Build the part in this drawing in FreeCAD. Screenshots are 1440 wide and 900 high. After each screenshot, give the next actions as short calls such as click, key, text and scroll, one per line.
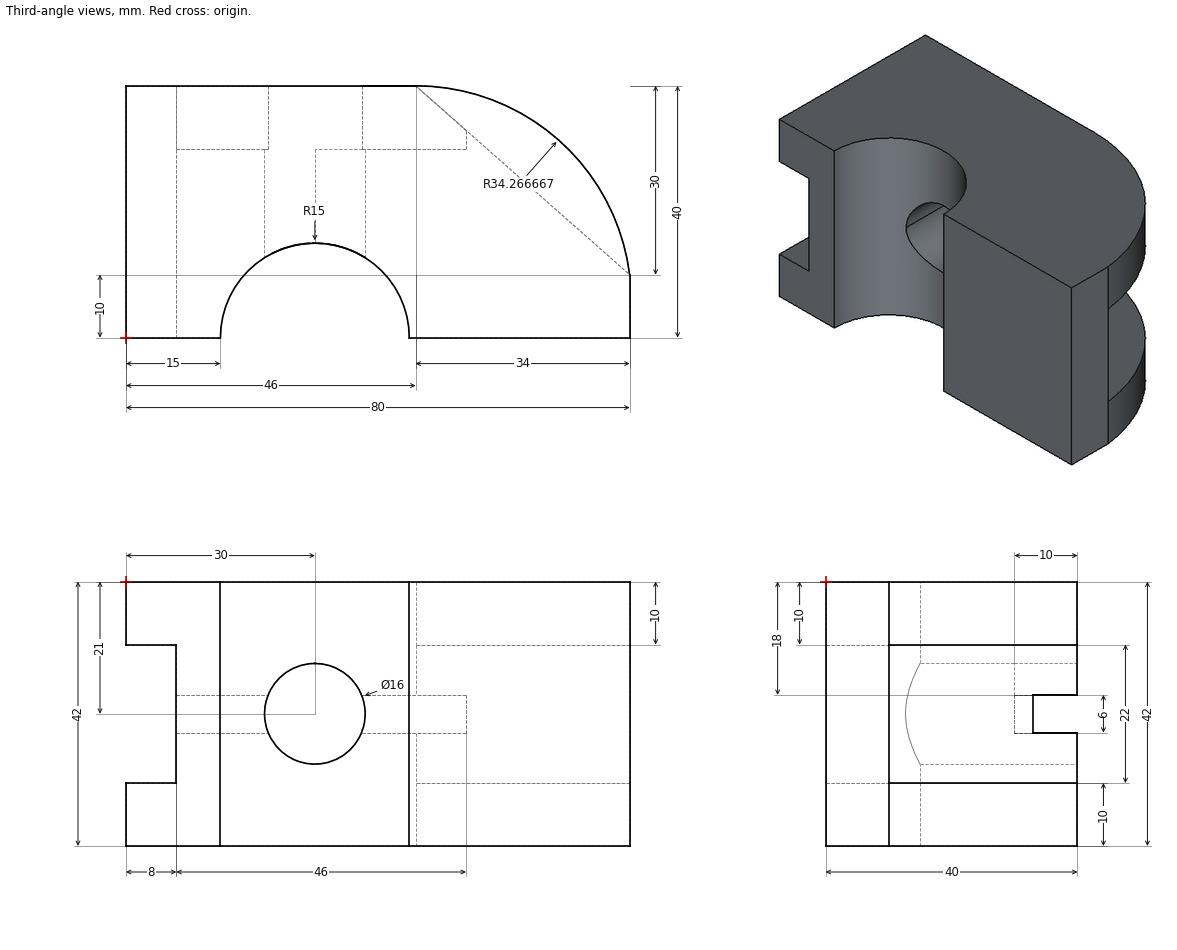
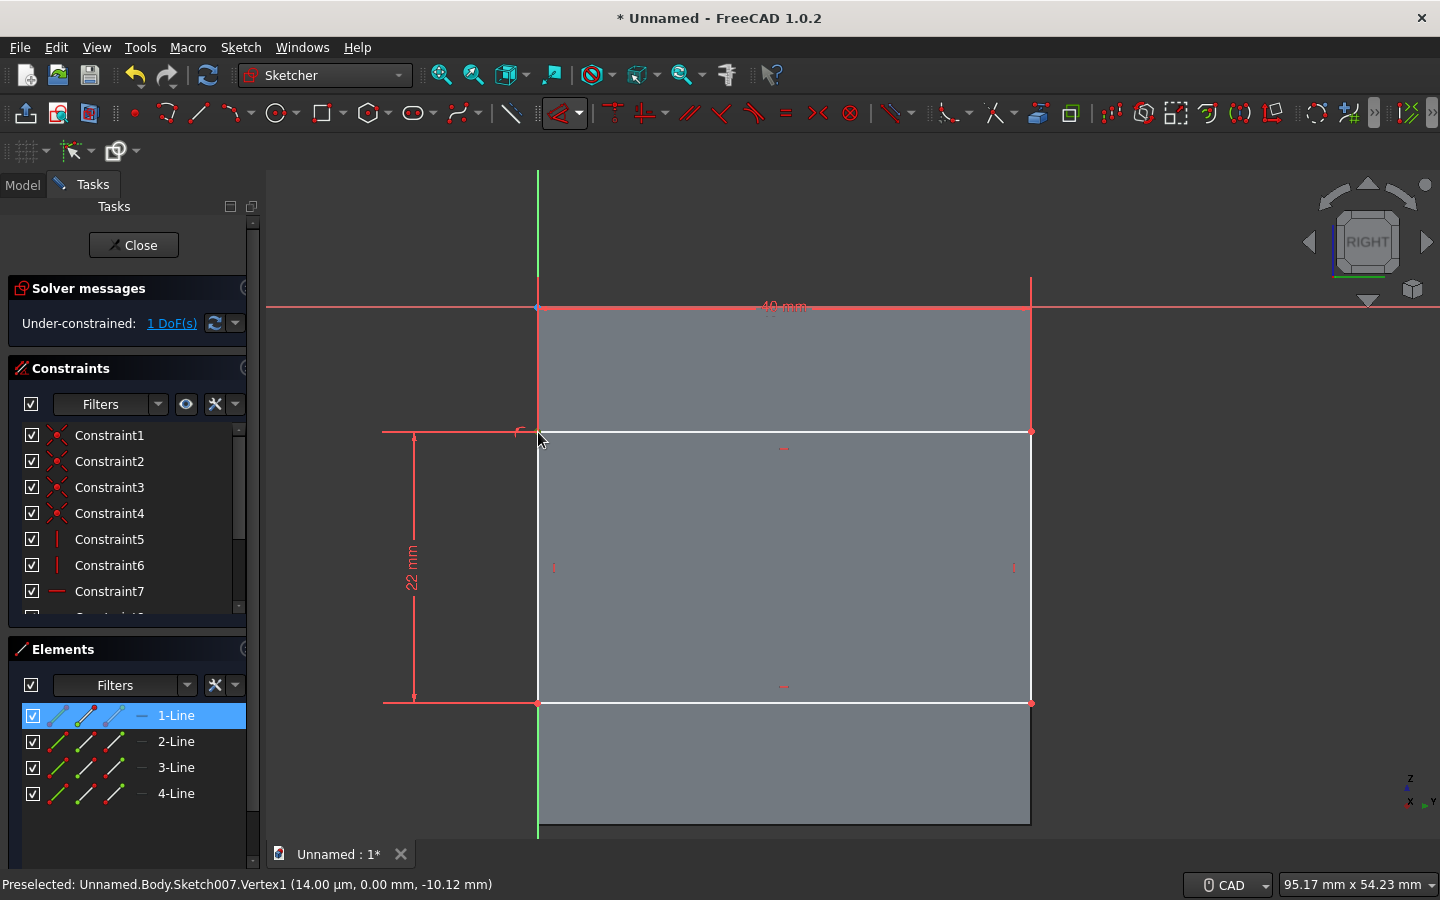
click(582, 114)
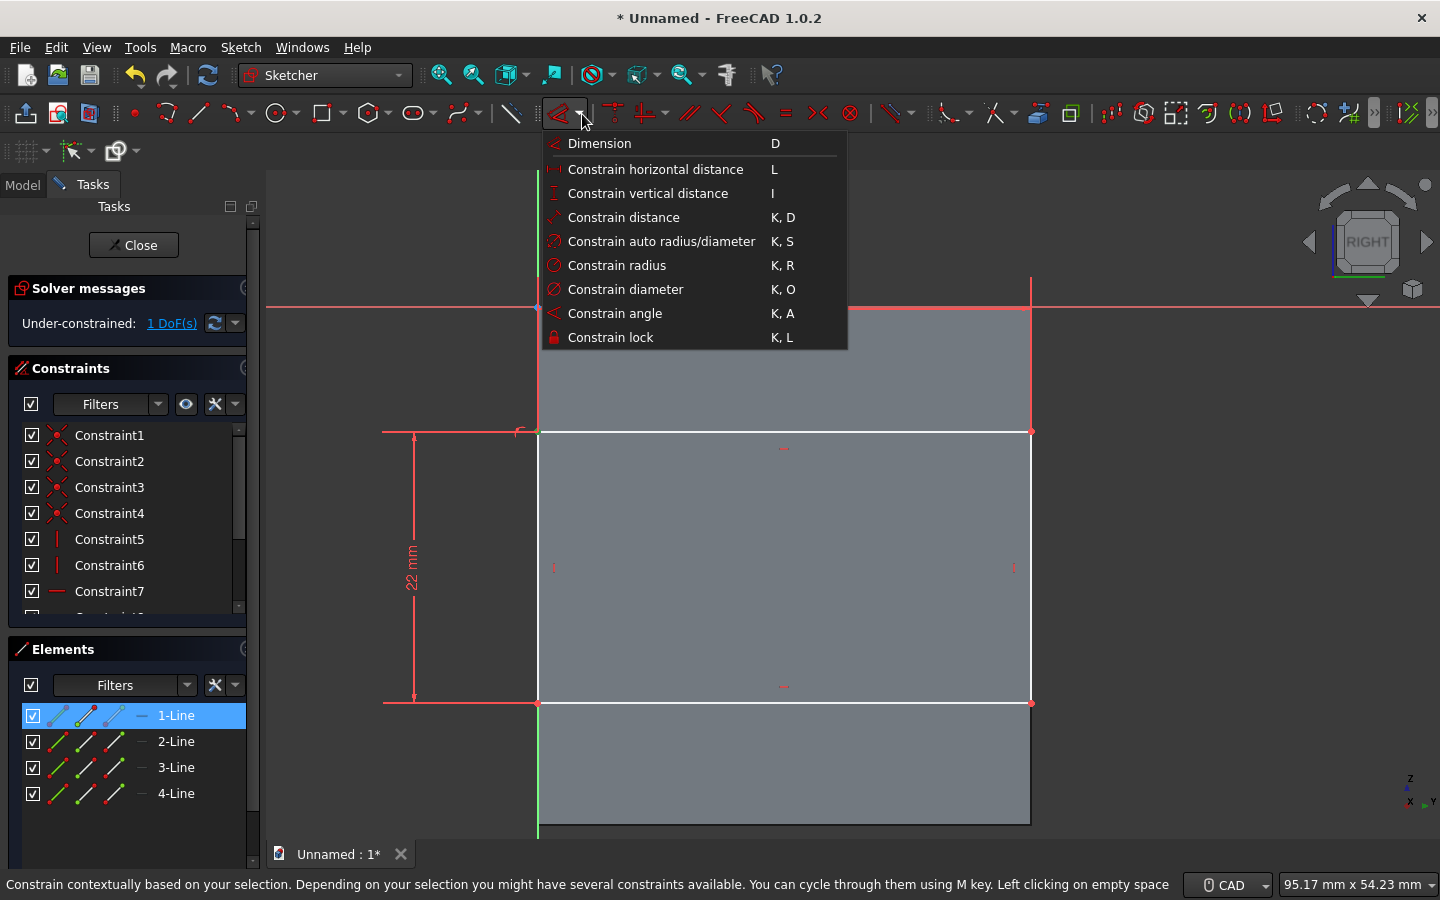
click(695, 193)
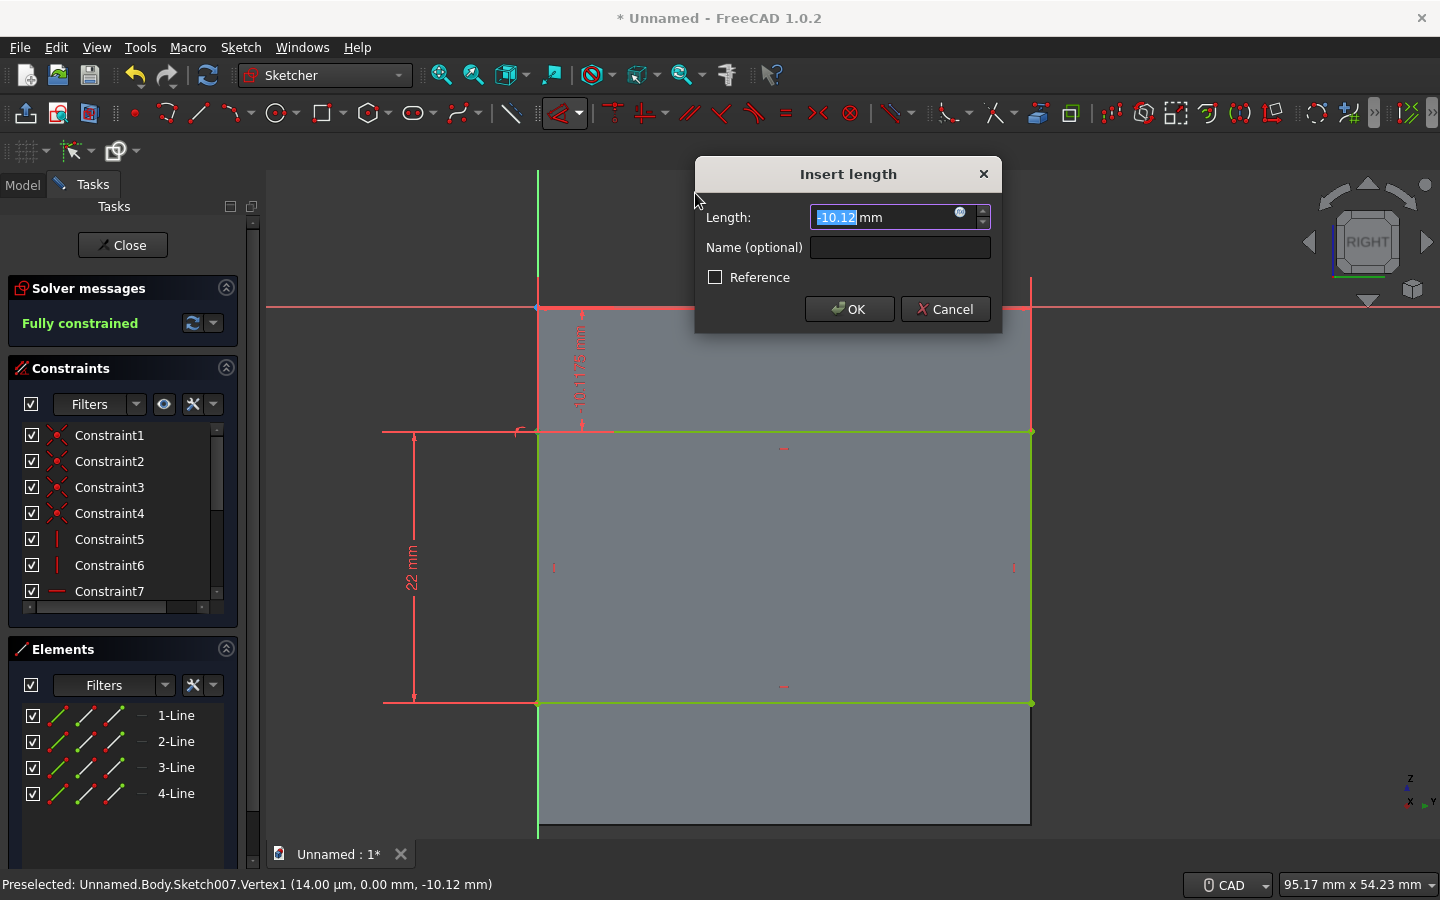
text(-10)
key(Return)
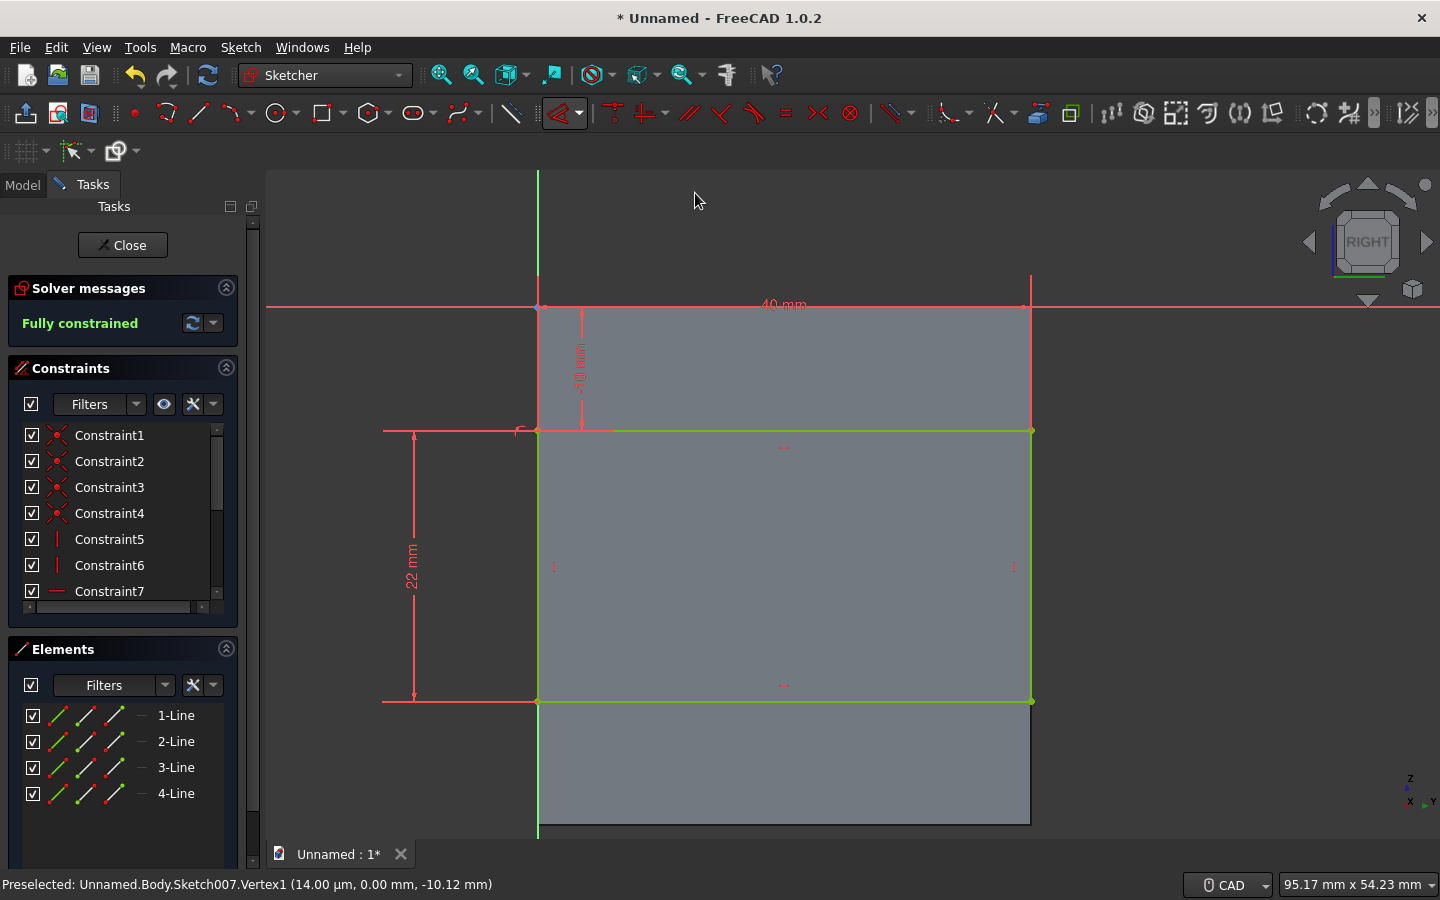
click(123, 245)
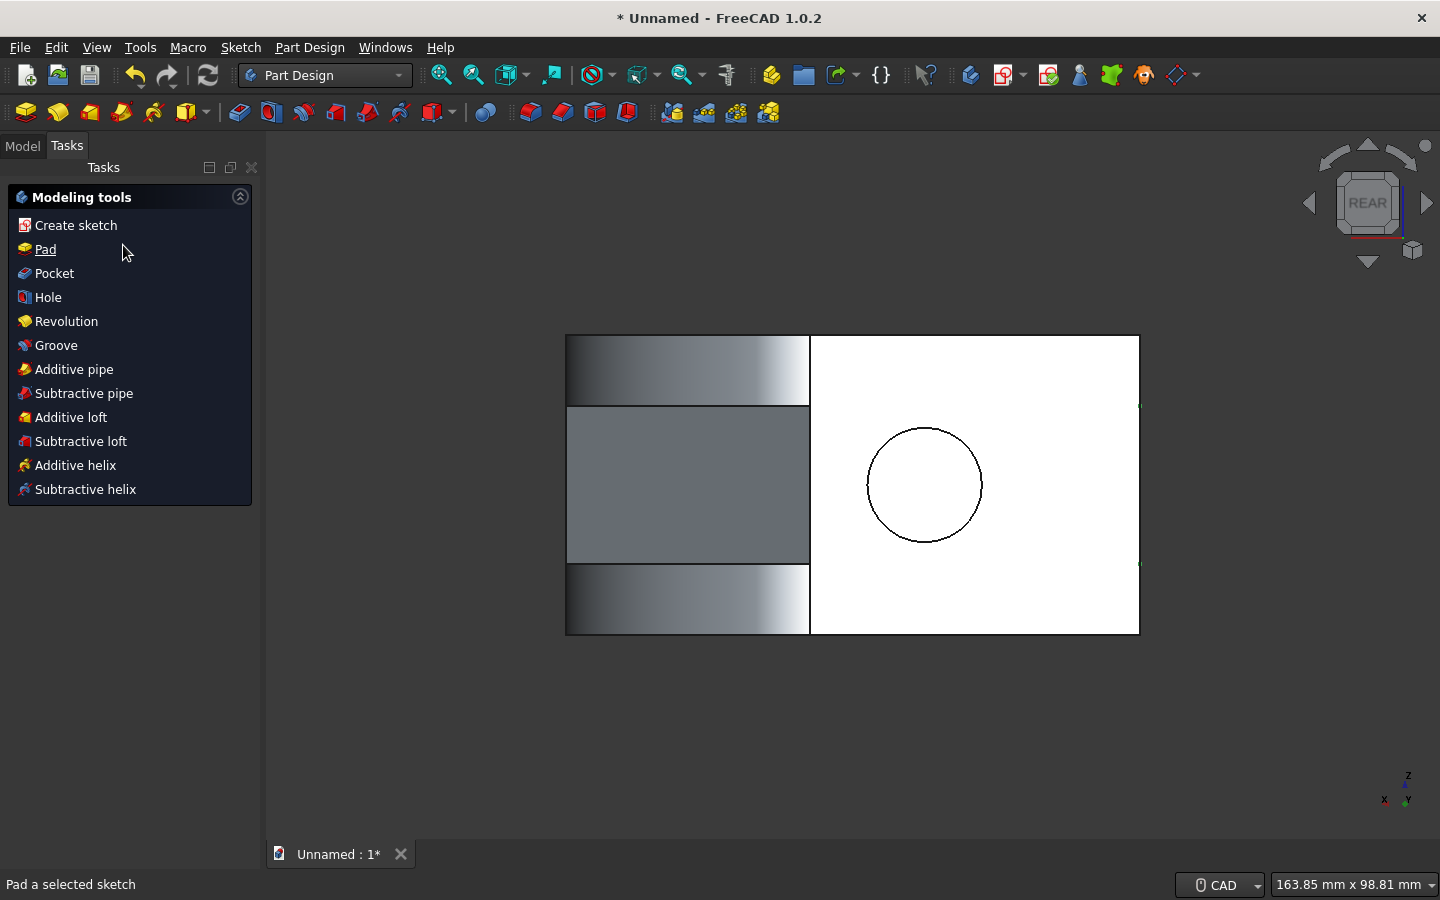
click(240, 112)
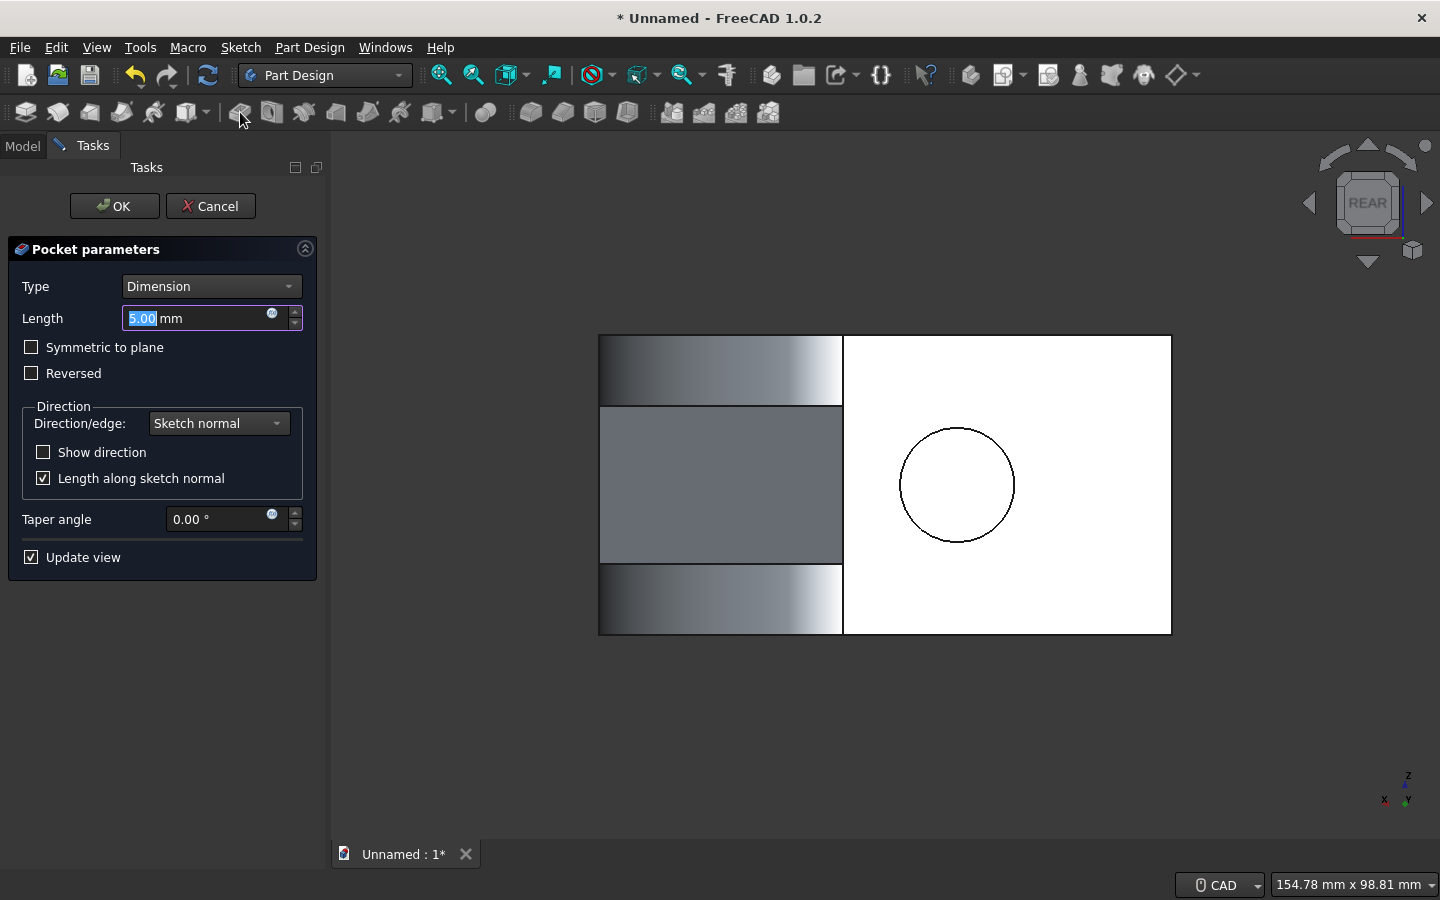
text(8)
key(Tab)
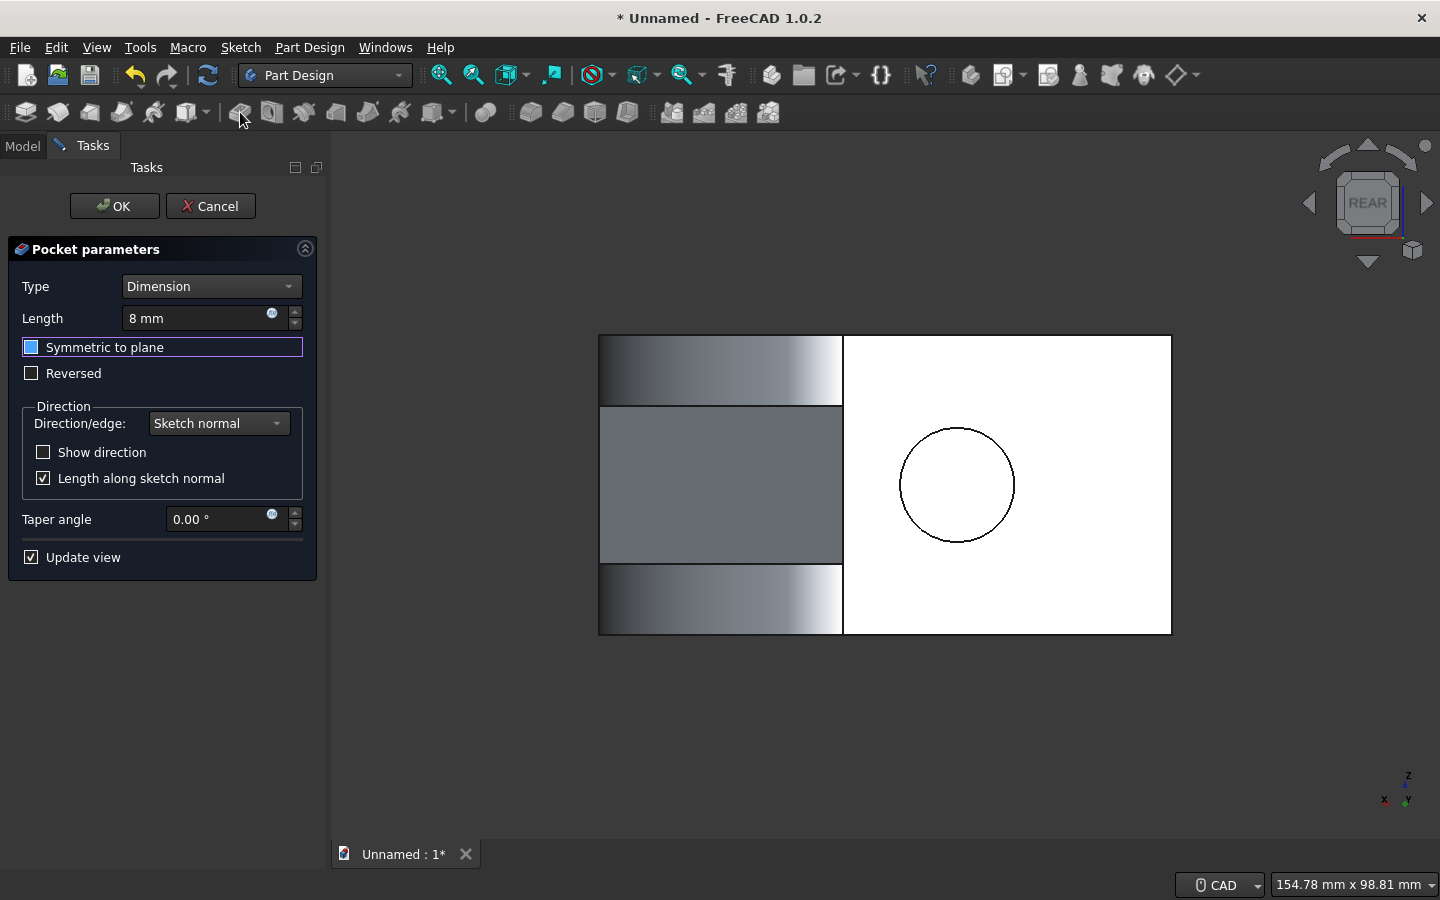
click(30, 373)